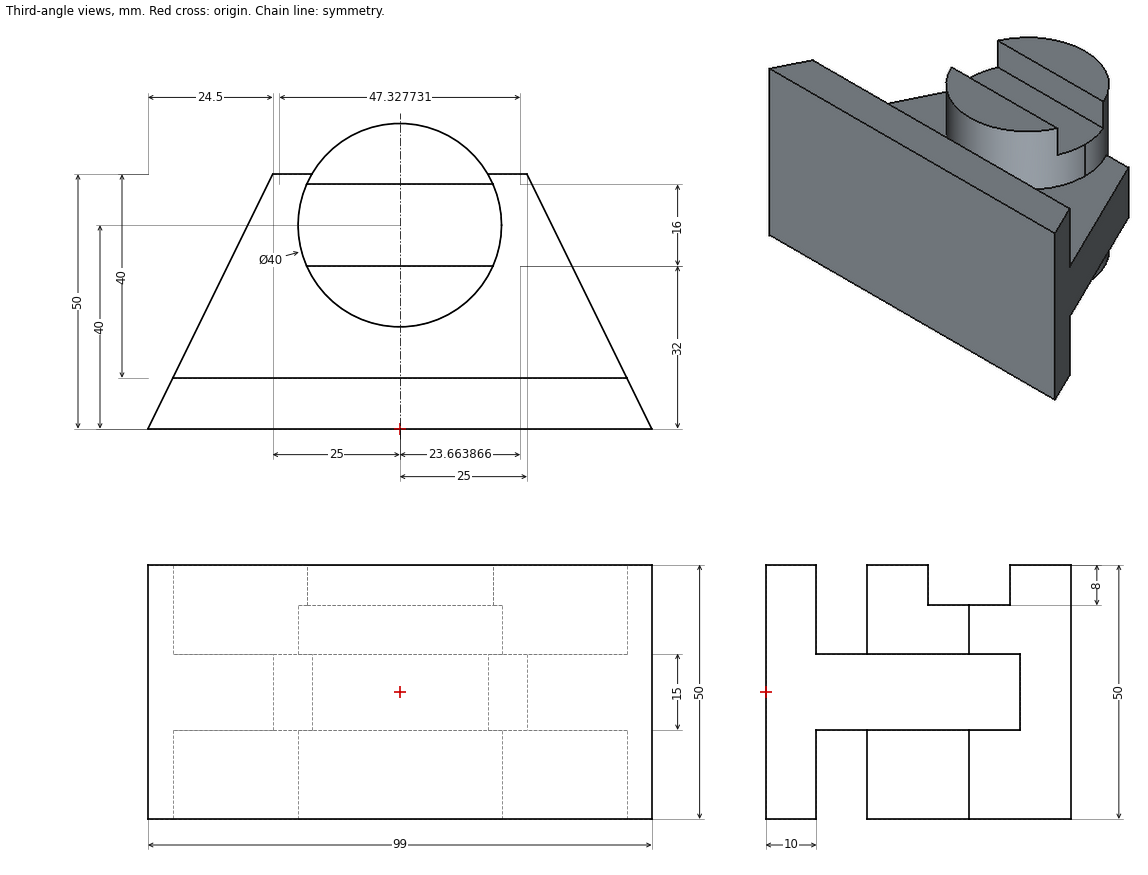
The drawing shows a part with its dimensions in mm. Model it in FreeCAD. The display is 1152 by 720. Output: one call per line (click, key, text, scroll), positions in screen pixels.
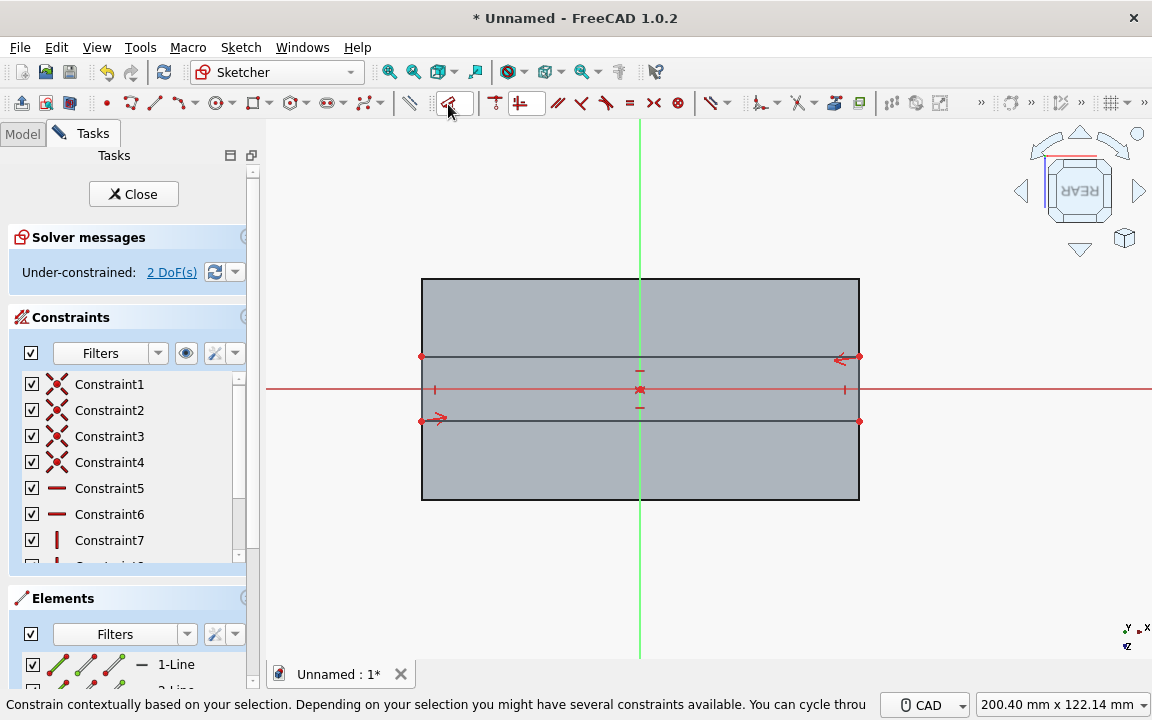
click(553, 421)
click(540, 455)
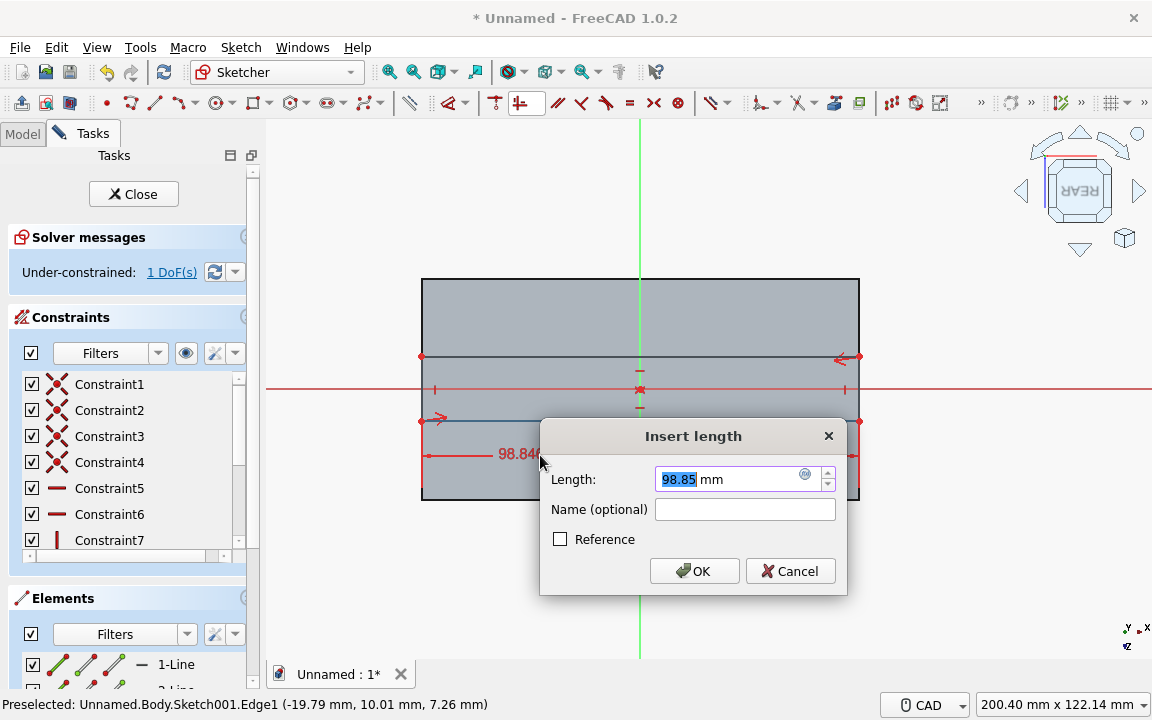
text(99)
key(Return)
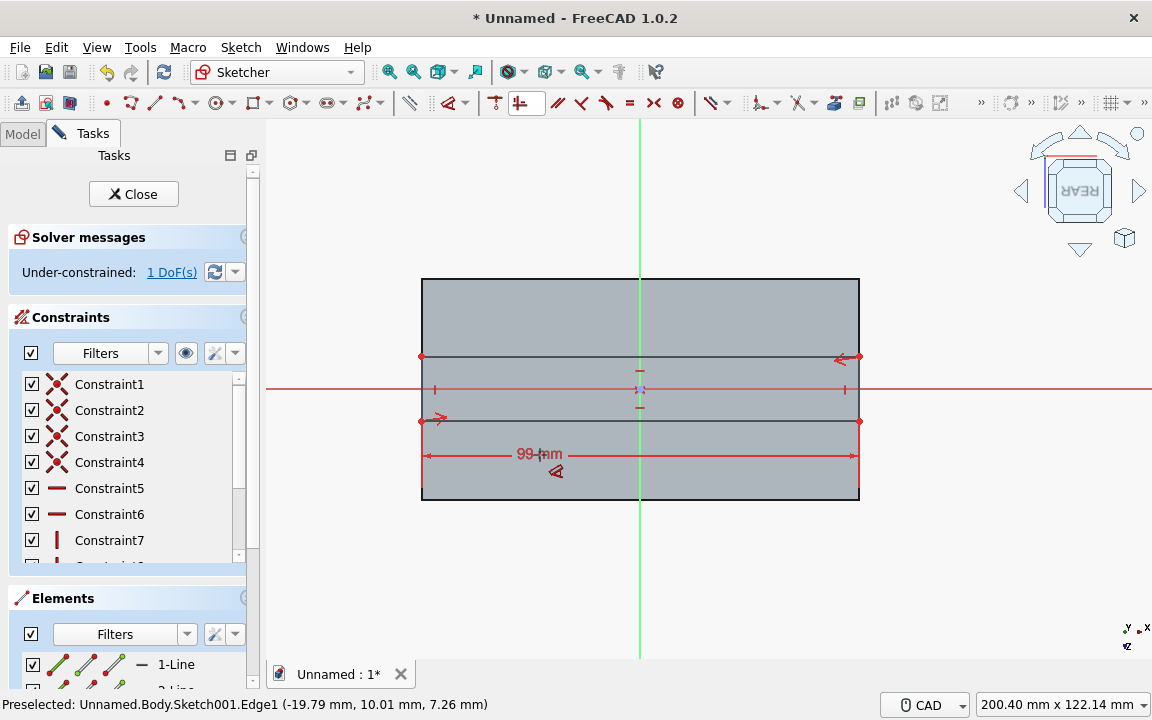
click(859, 402)
click(893, 374)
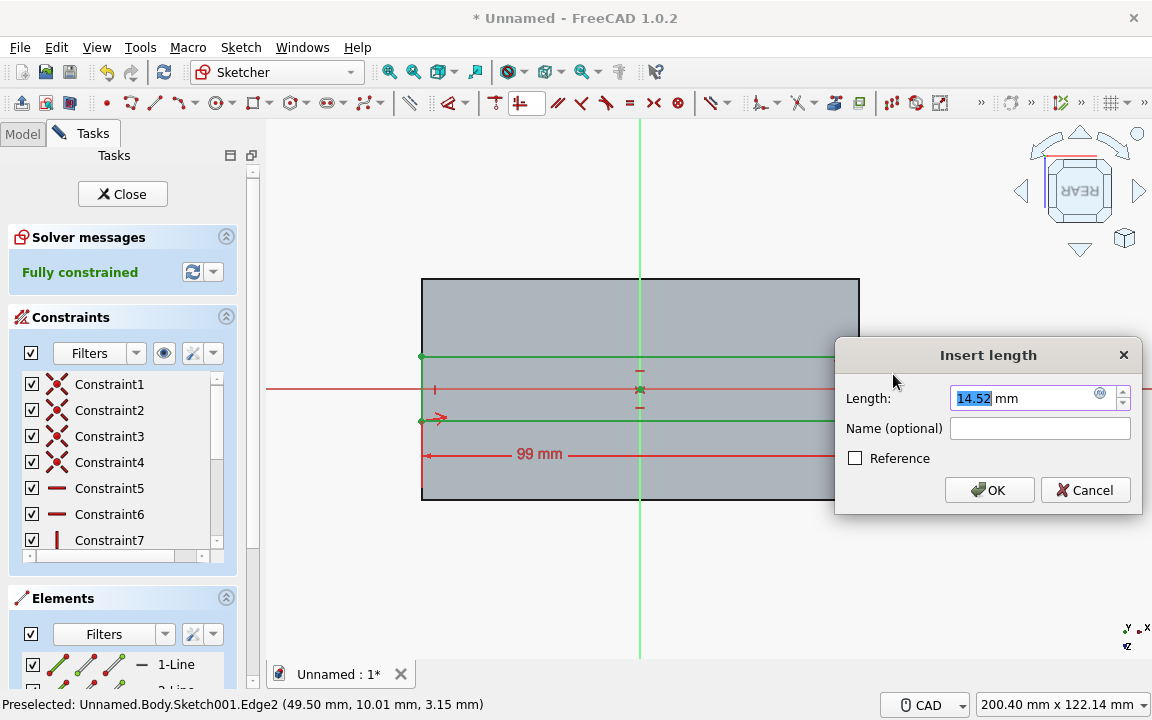
text(15)
key(Return)
key(Escape)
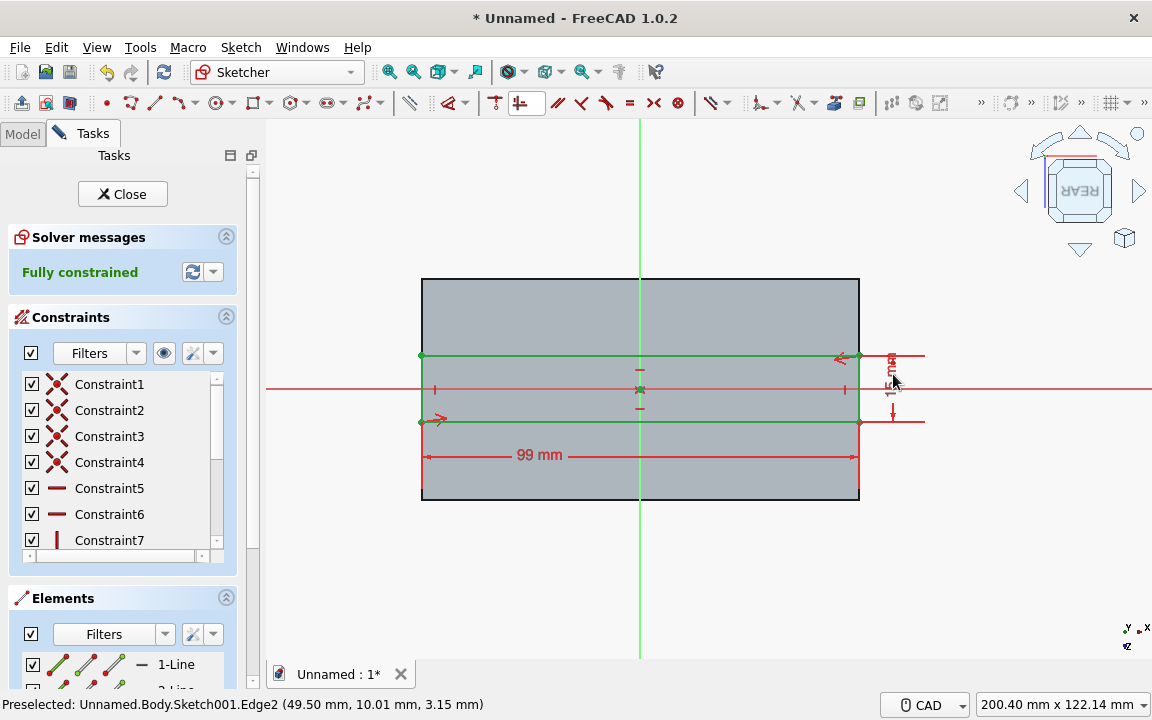
click(123, 194)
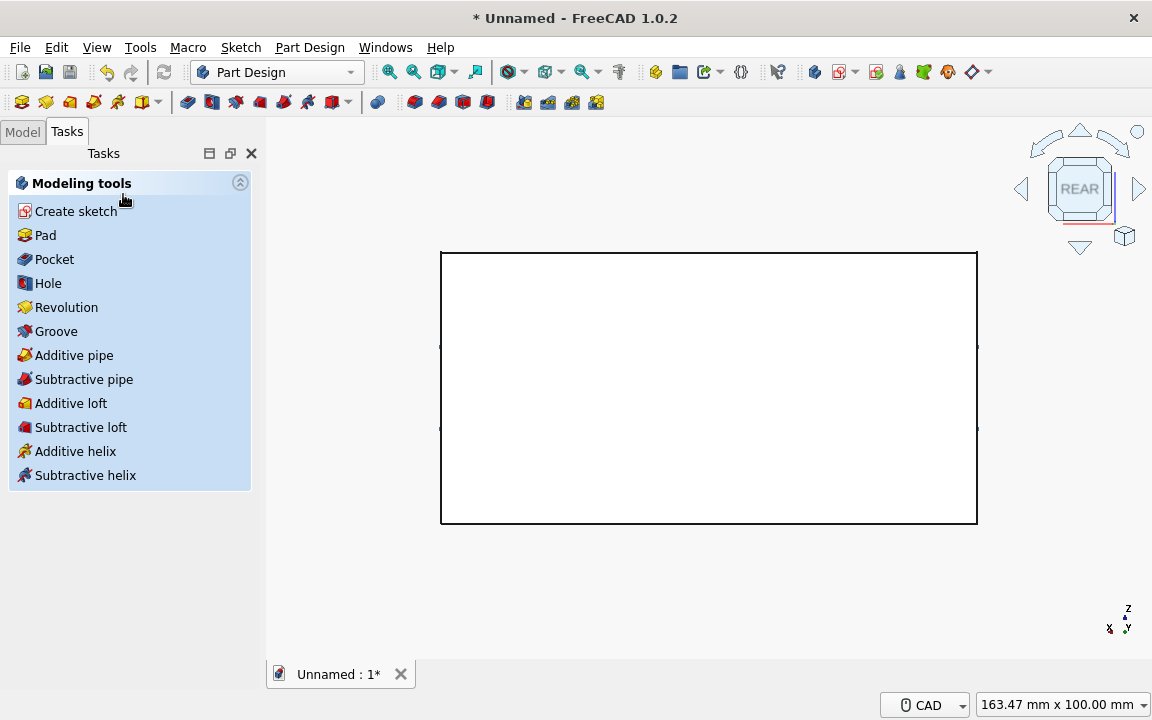
click(22, 102)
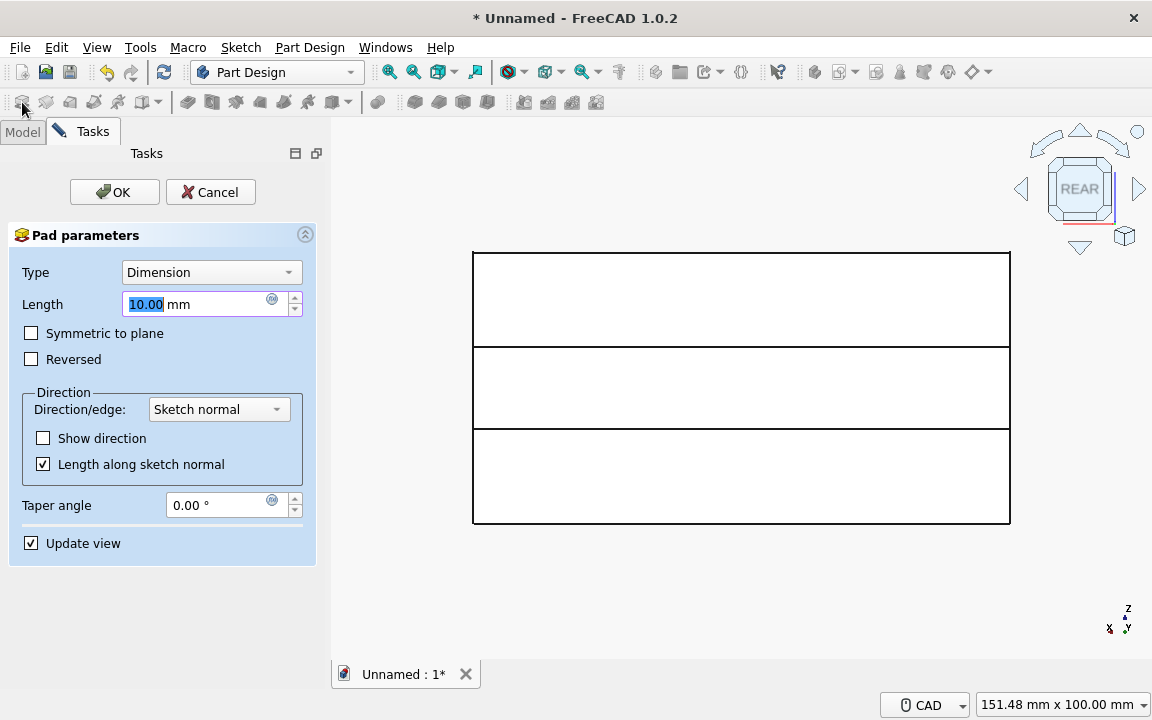
text(40)
key(Tab)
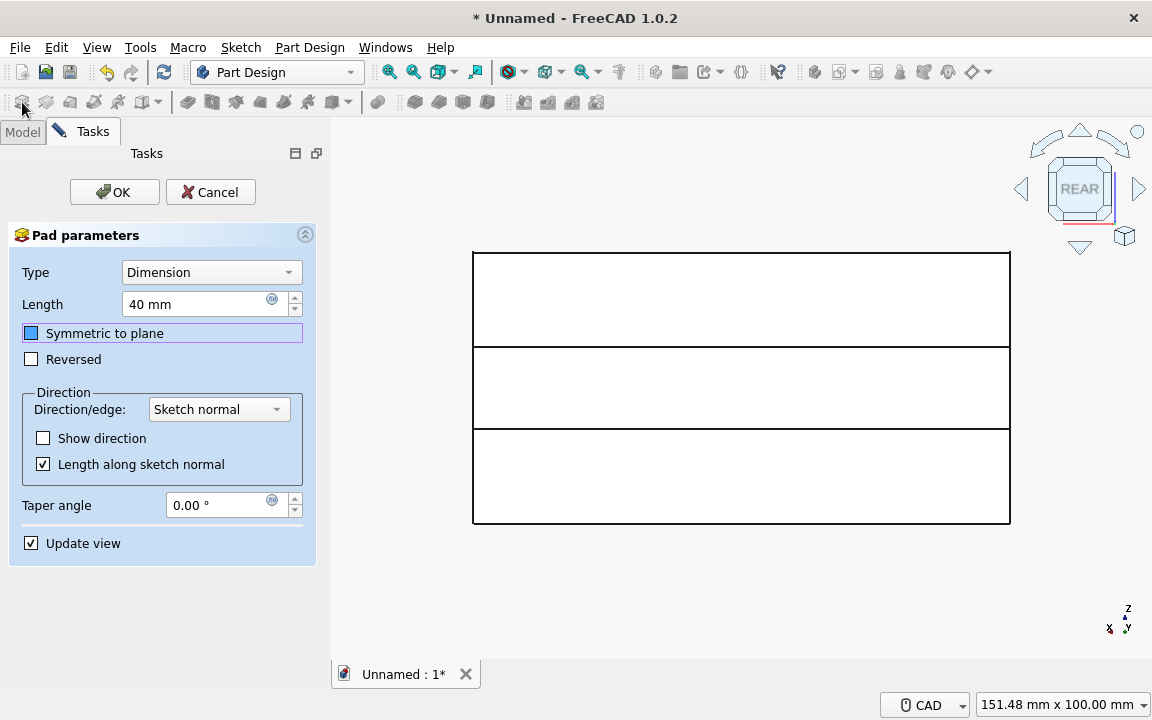
click(115, 192)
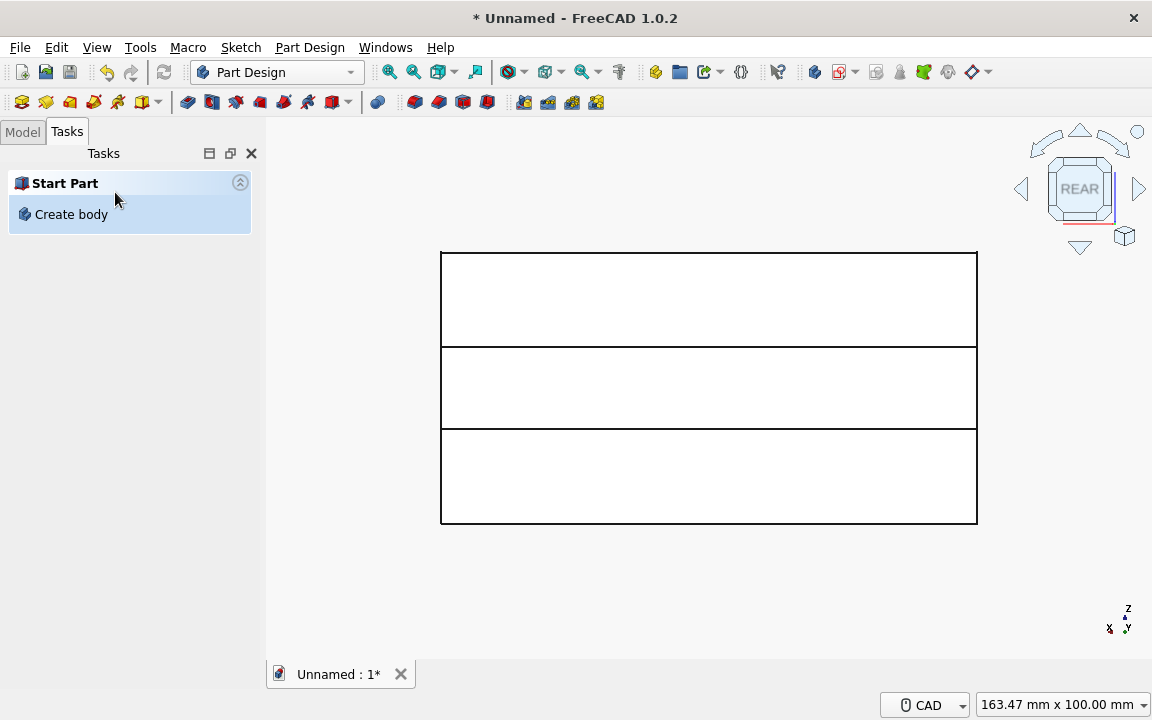
click(840, 72)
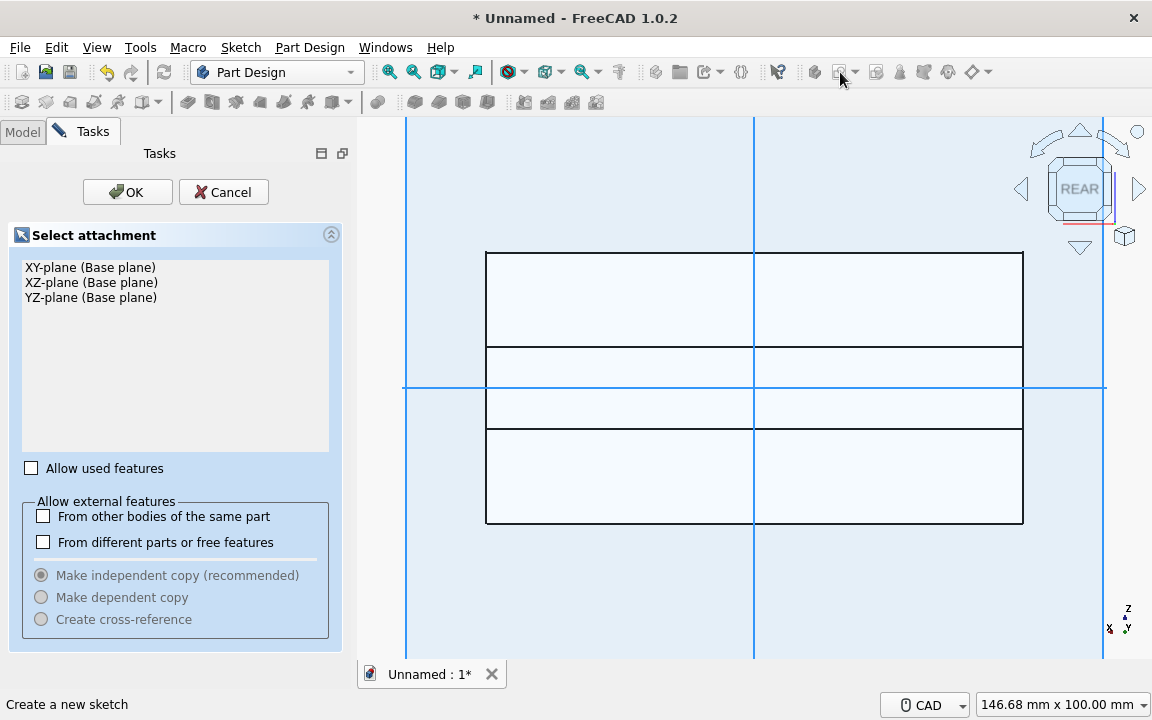
click(82, 268)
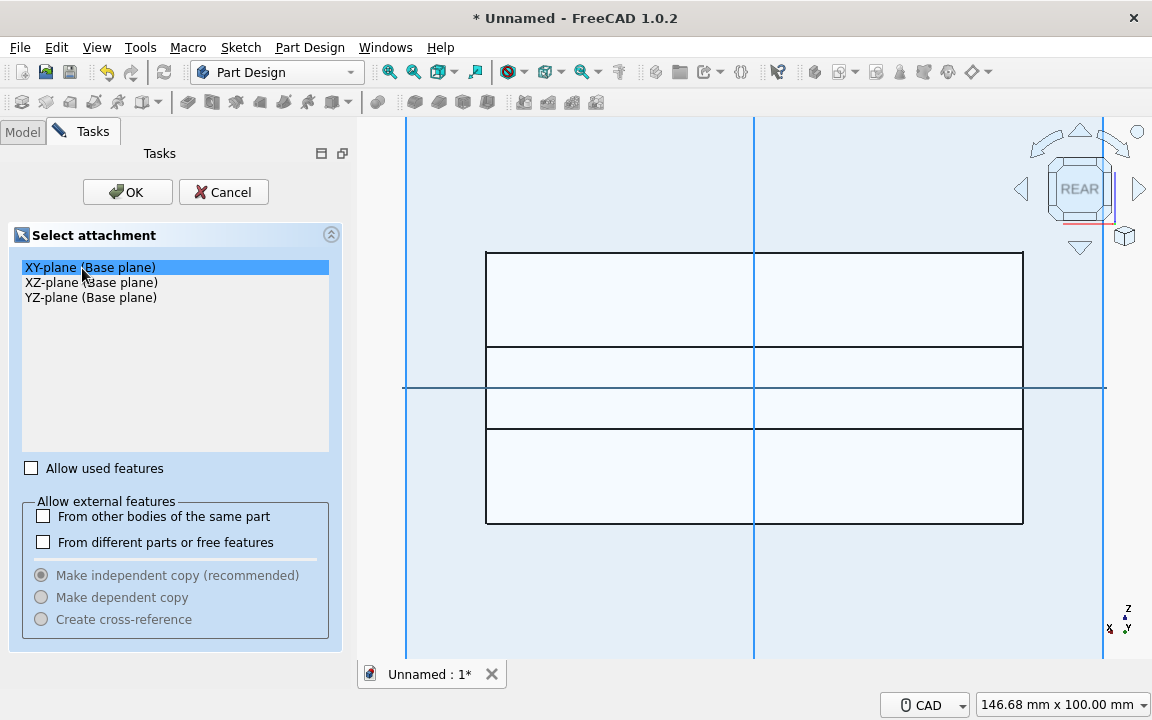
click(128, 192)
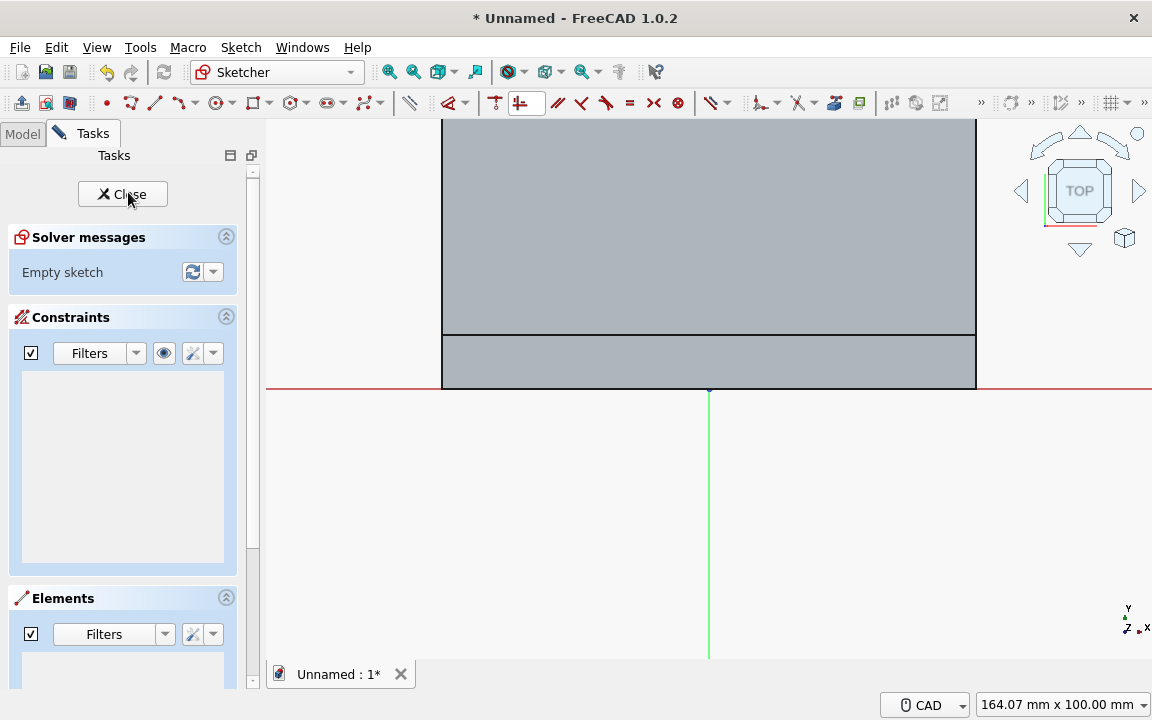
click(70, 104)